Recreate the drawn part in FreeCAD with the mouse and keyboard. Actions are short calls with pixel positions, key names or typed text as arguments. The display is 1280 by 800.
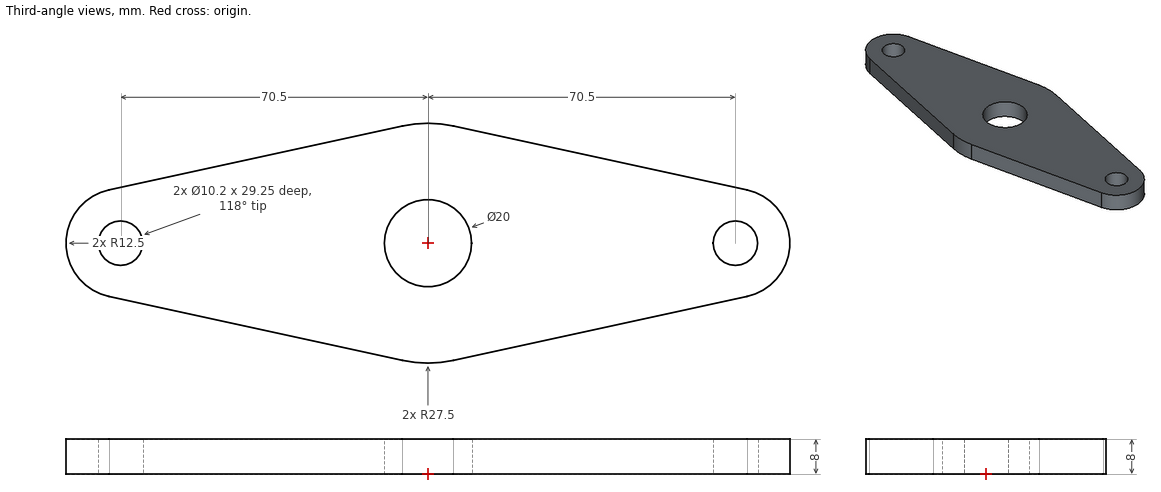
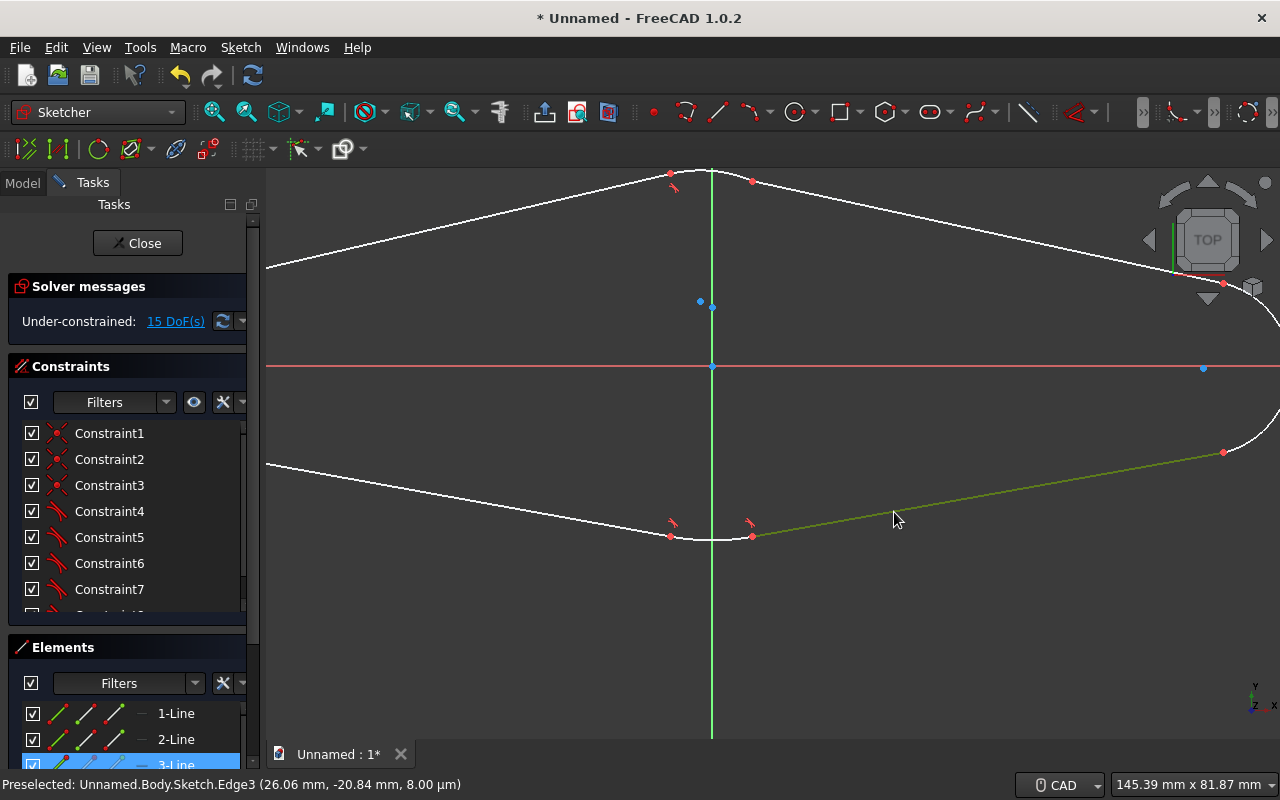
scroll(695, 560, down, 3)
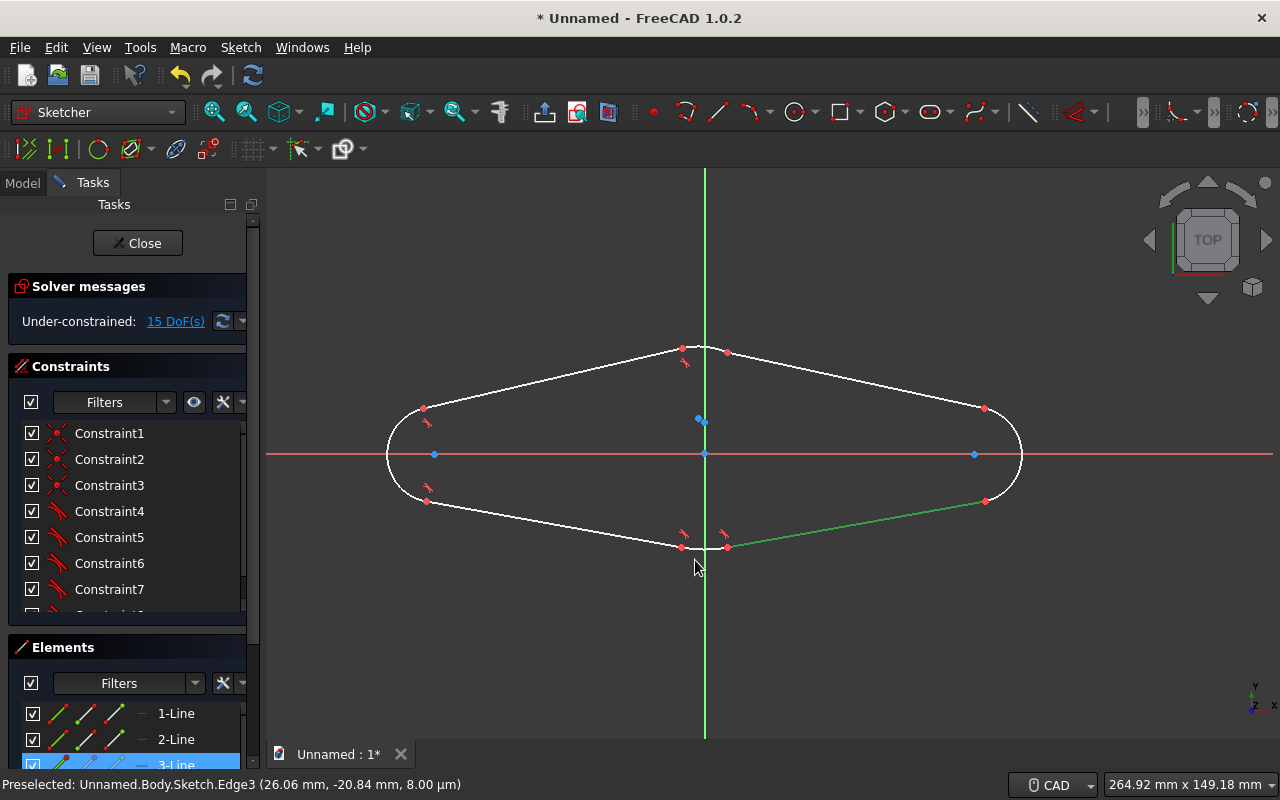
click(1015, 479)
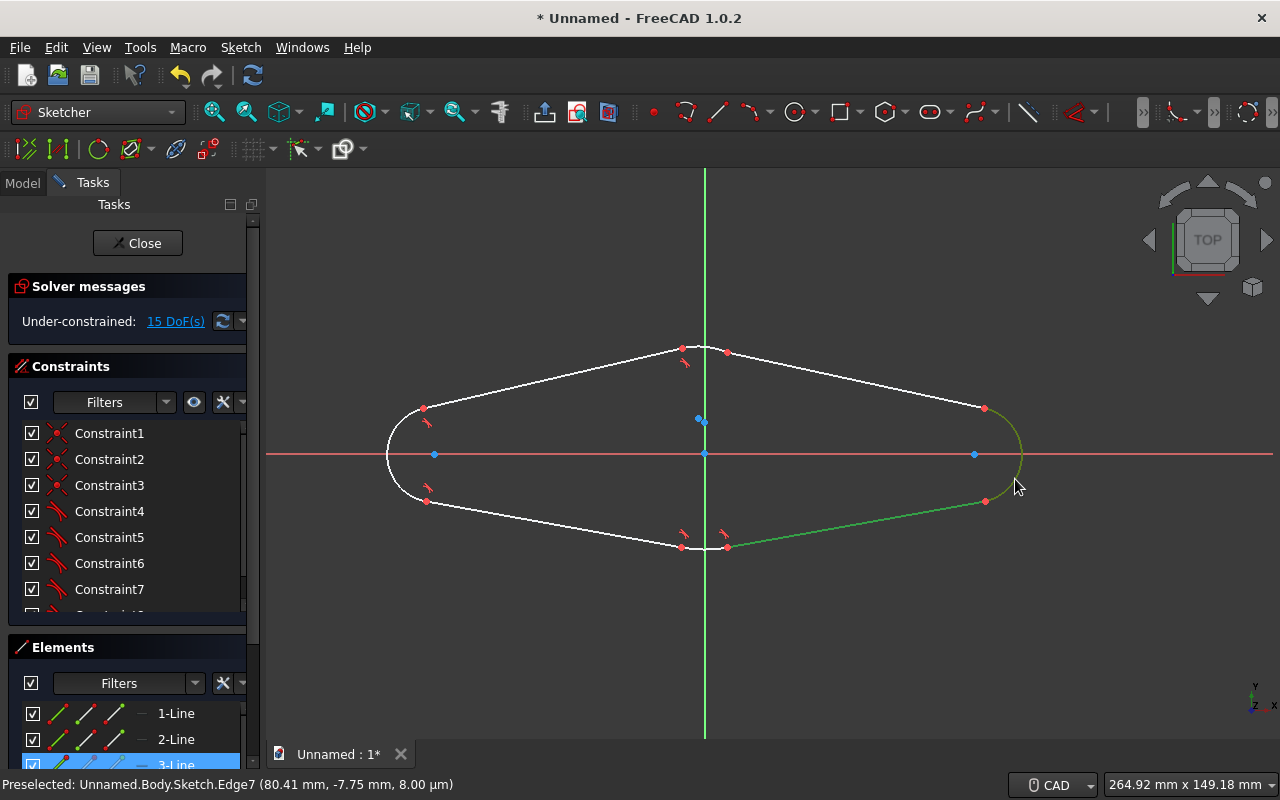
key(t)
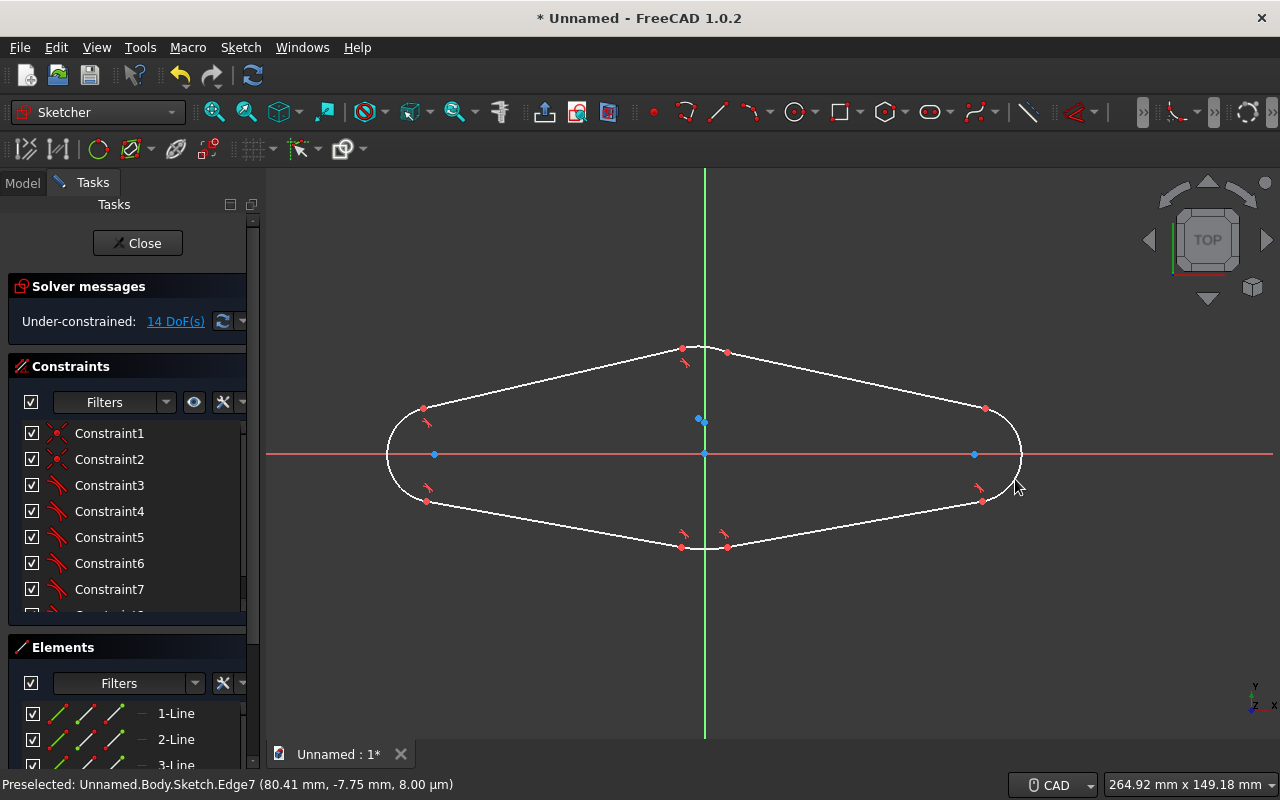
click(908, 392)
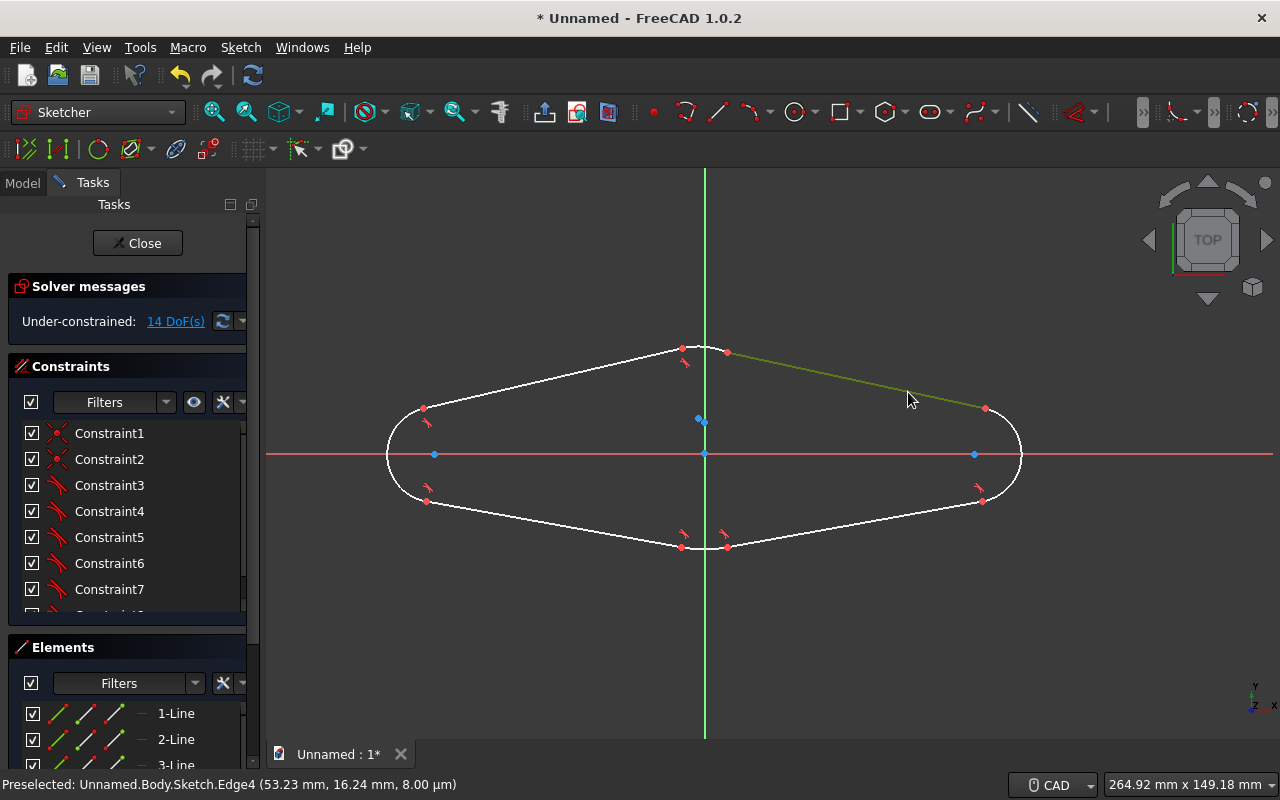
click(1014, 480)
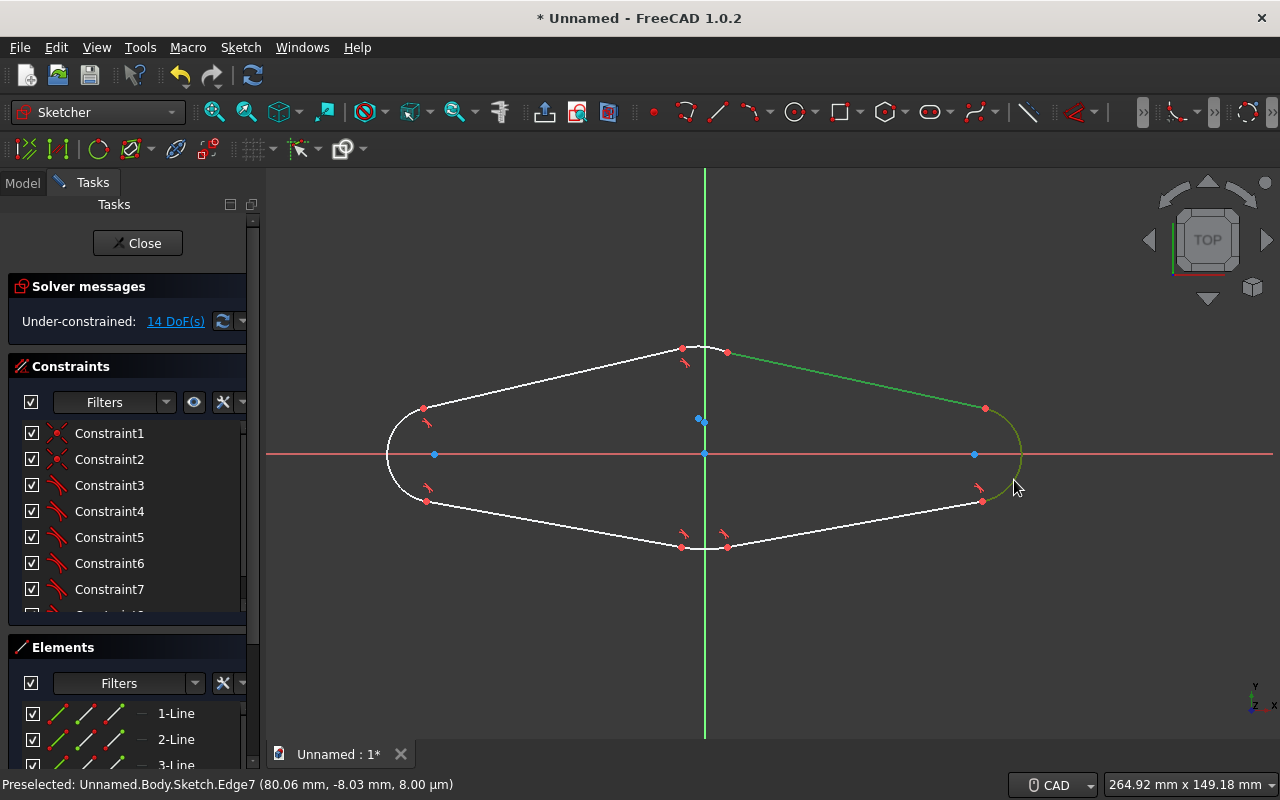
key(t)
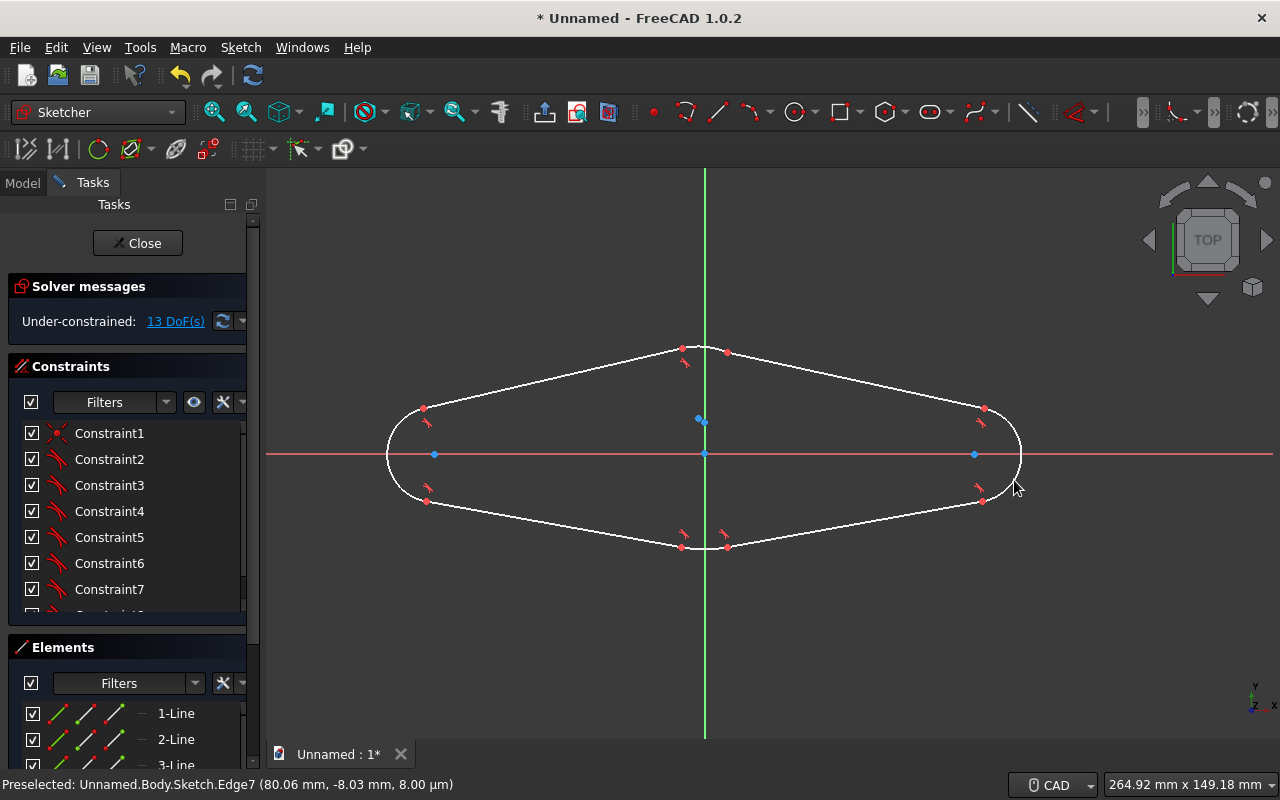
click(907, 392)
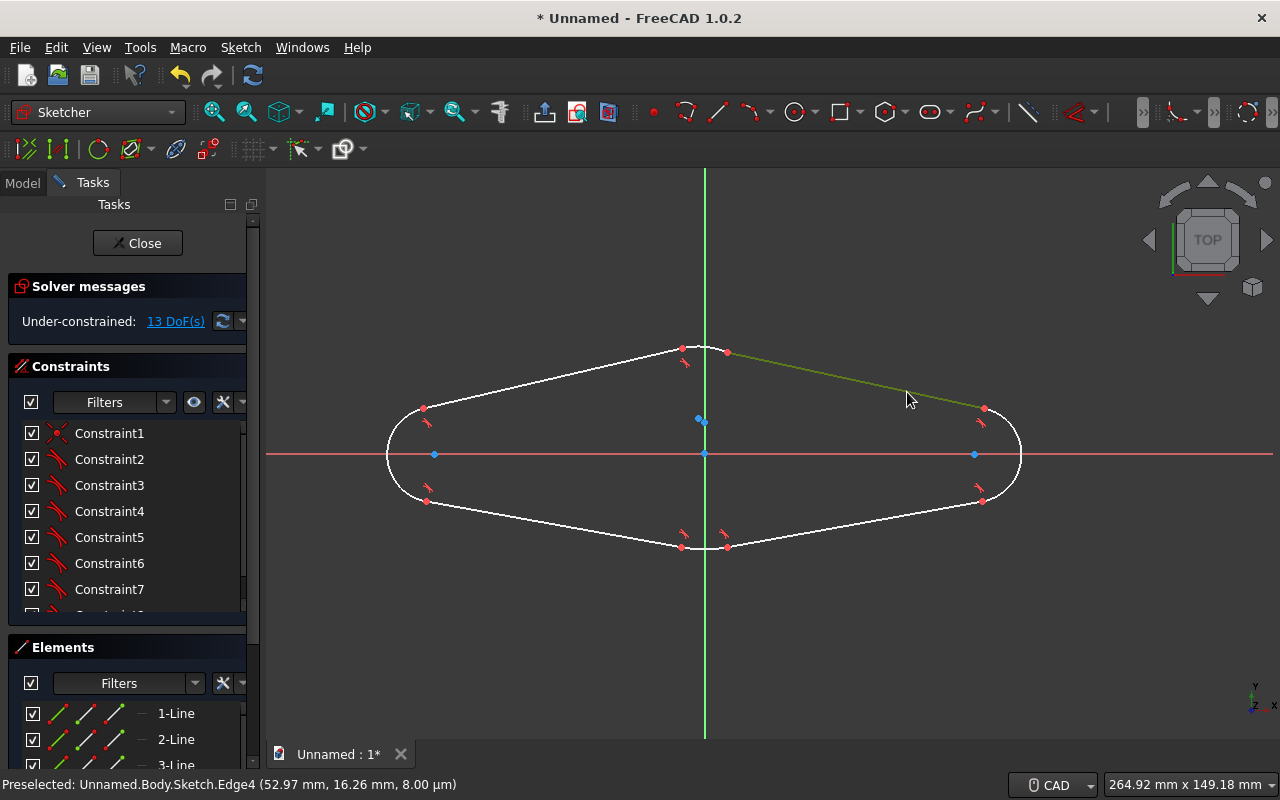
scroll(714, 348, up, 2)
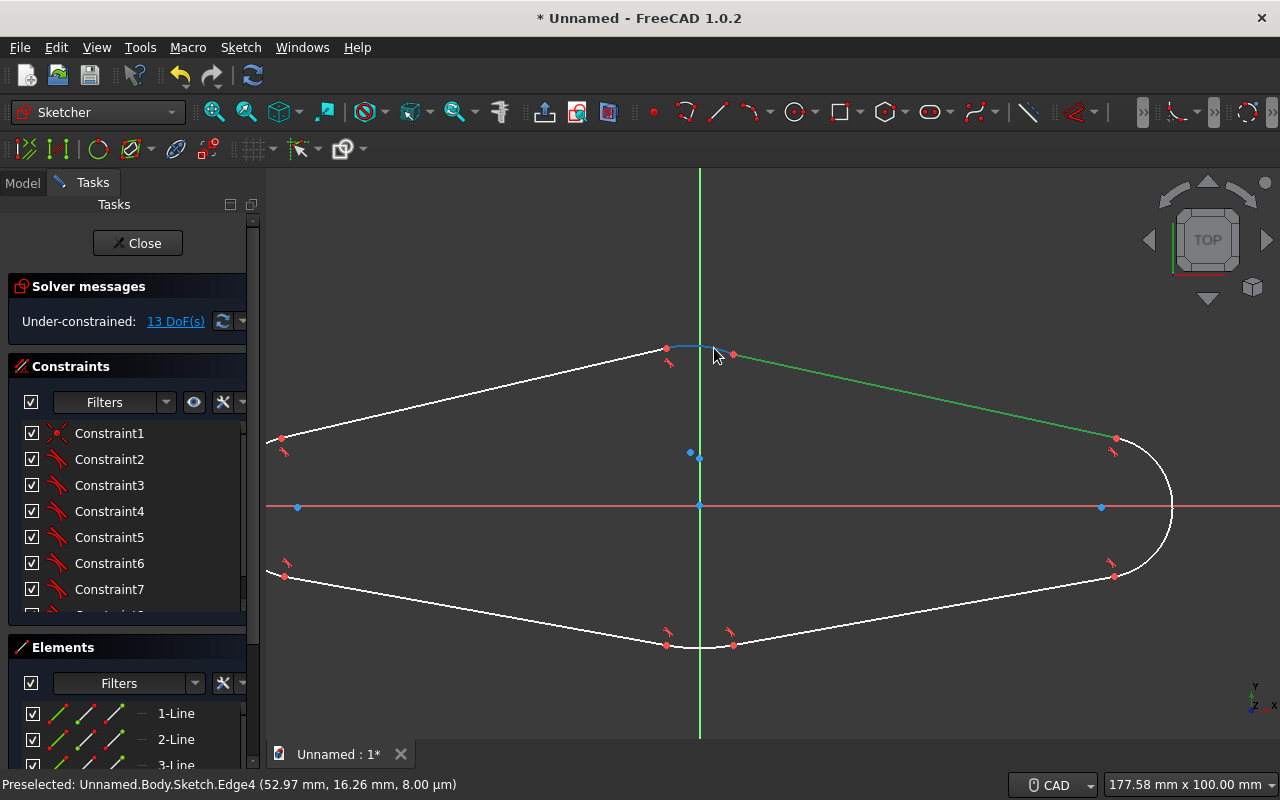
click(714, 348)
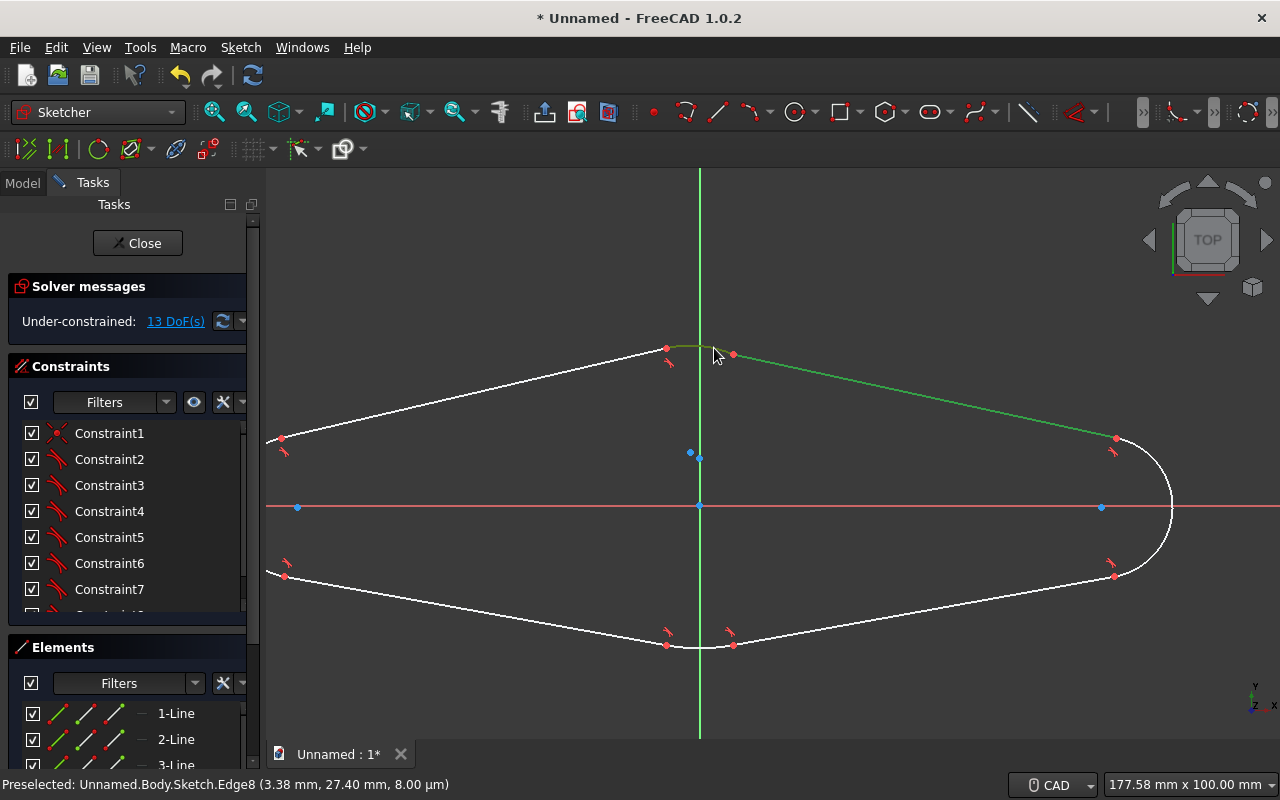
key(t)